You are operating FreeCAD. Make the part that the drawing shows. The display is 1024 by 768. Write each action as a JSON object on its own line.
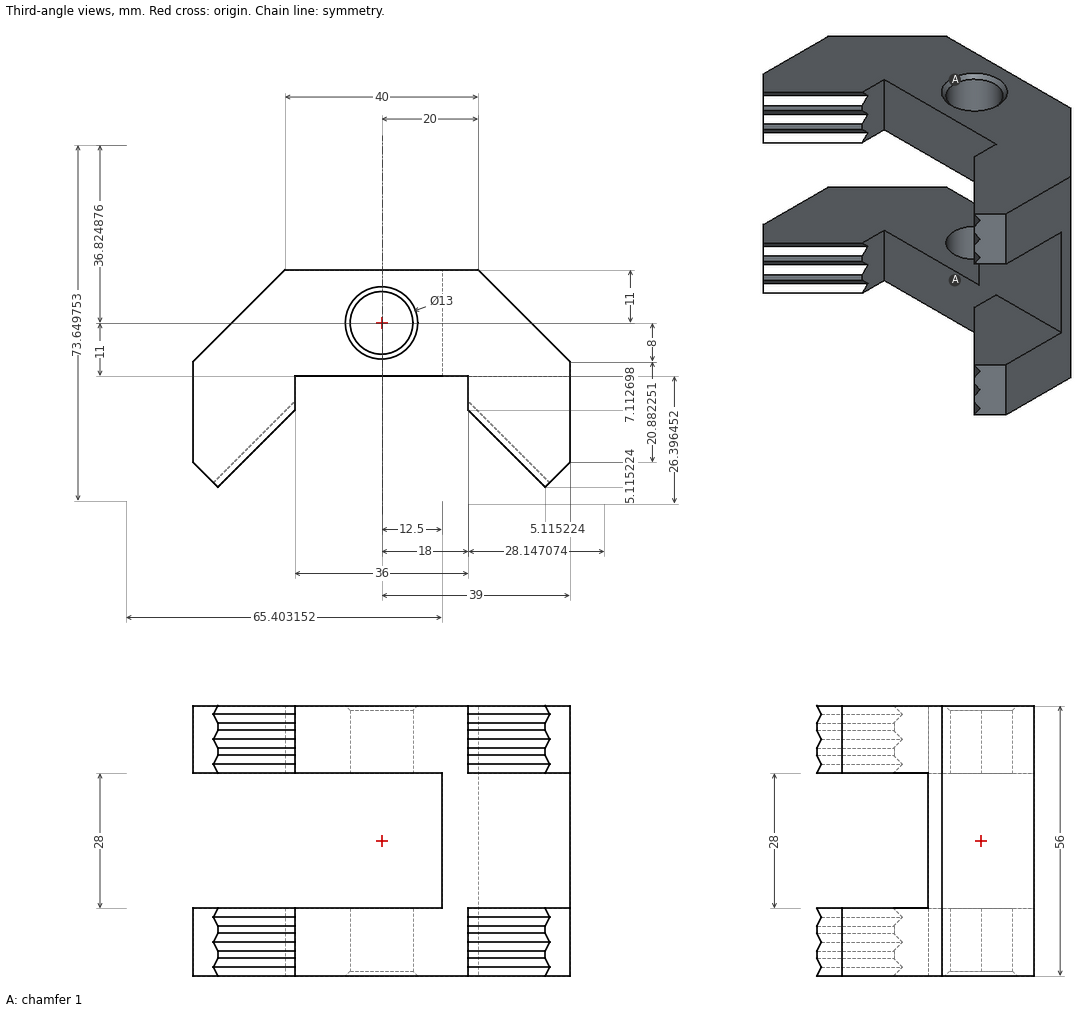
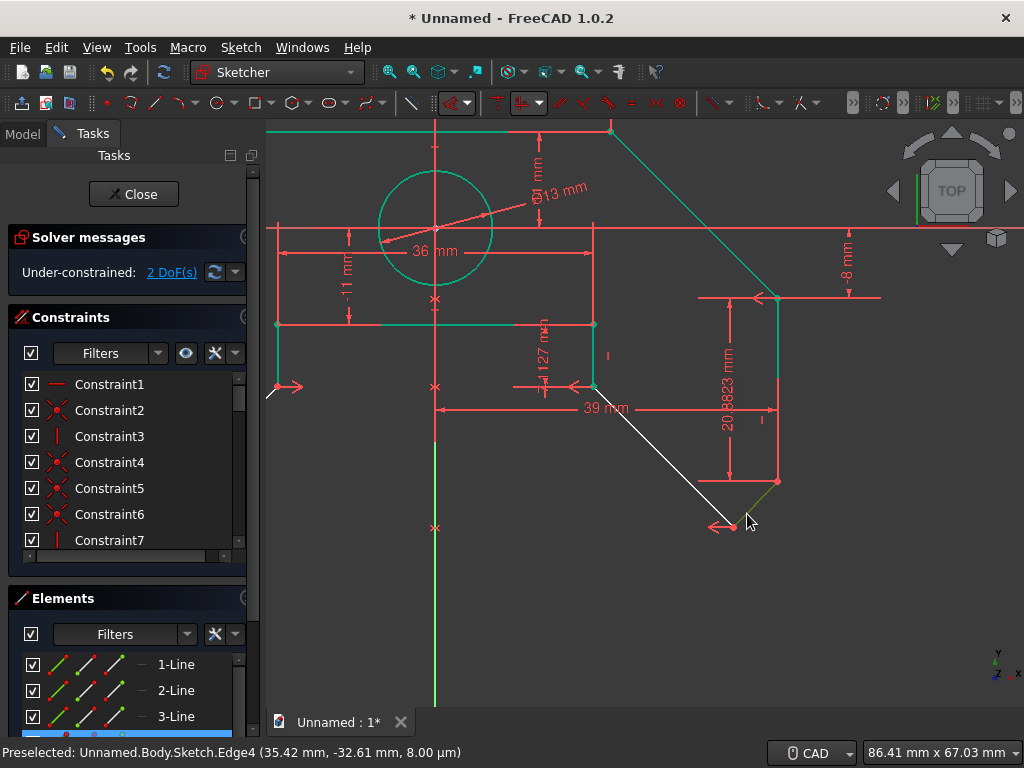
{"action": "key", "text": "l"}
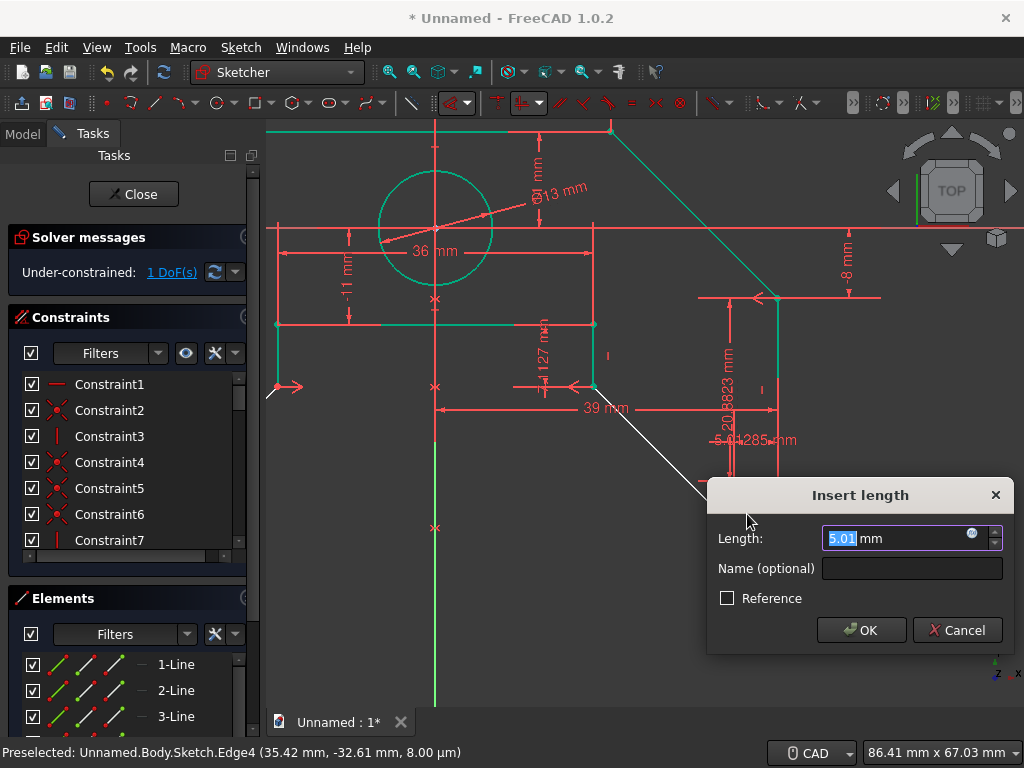
{"action": "type", "text": "5.115224"}
{"action": "key", "text": "Return"}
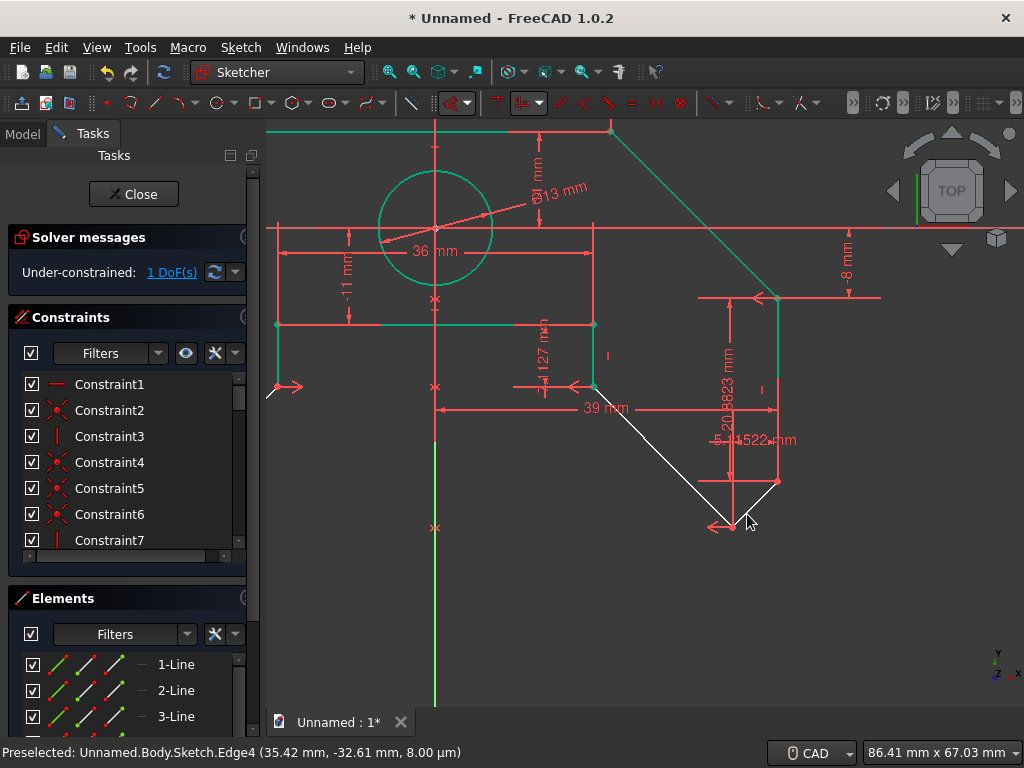
{"action": "left_click", "coordinate": [746, 514]}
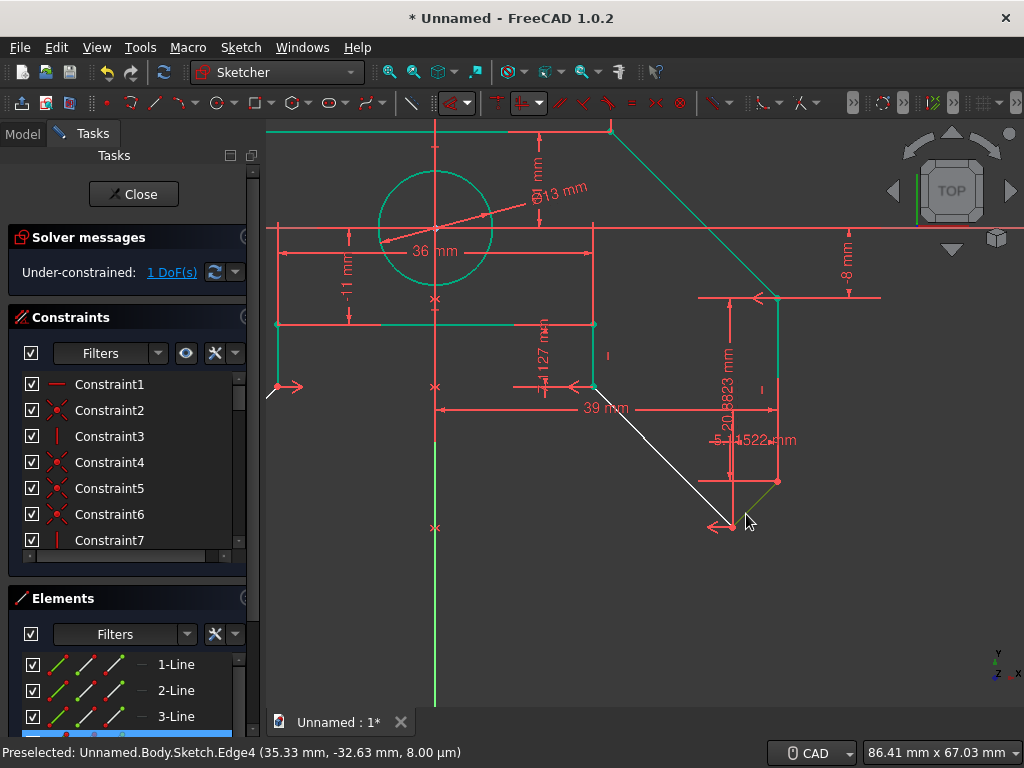
{"action": "left_click", "coordinate": [470, 104]}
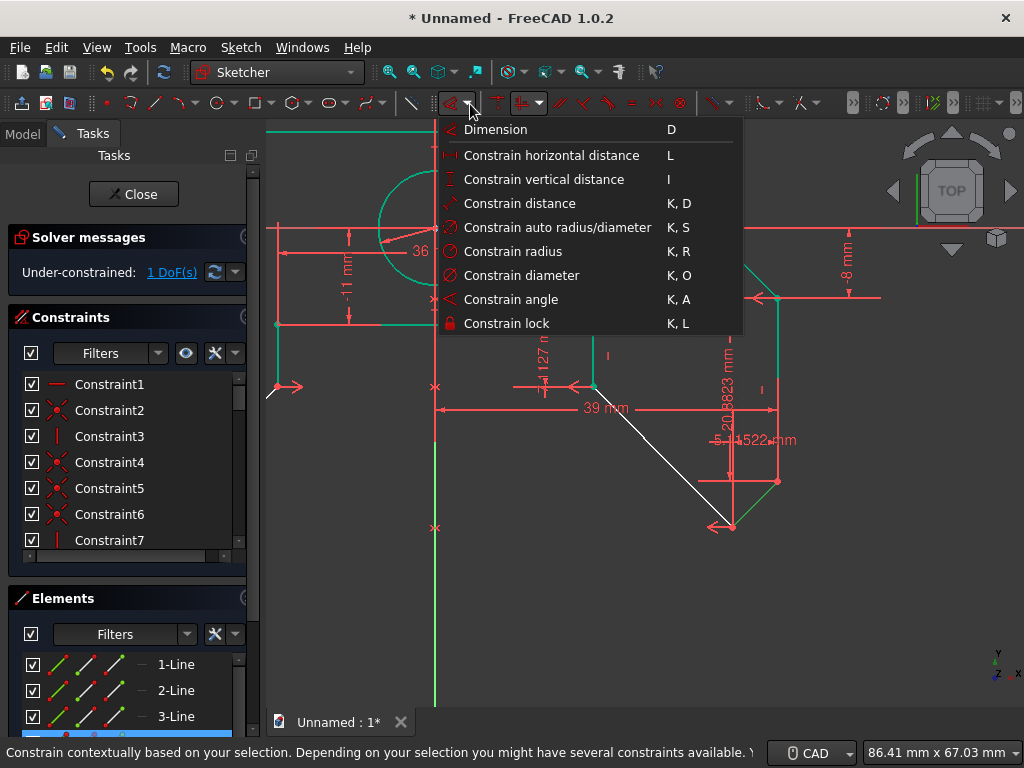
{"action": "left_click", "coordinate": [591, 179]}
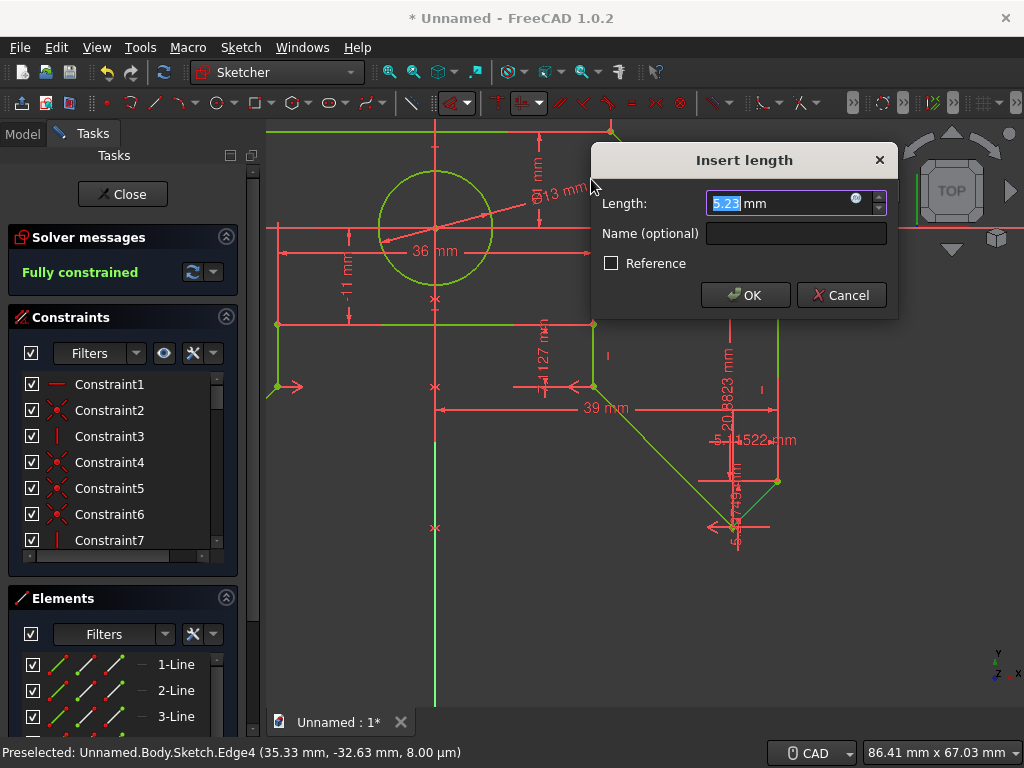
{"action": "type", "text": "5.115224"}
{"action": "key", "text": "Return"}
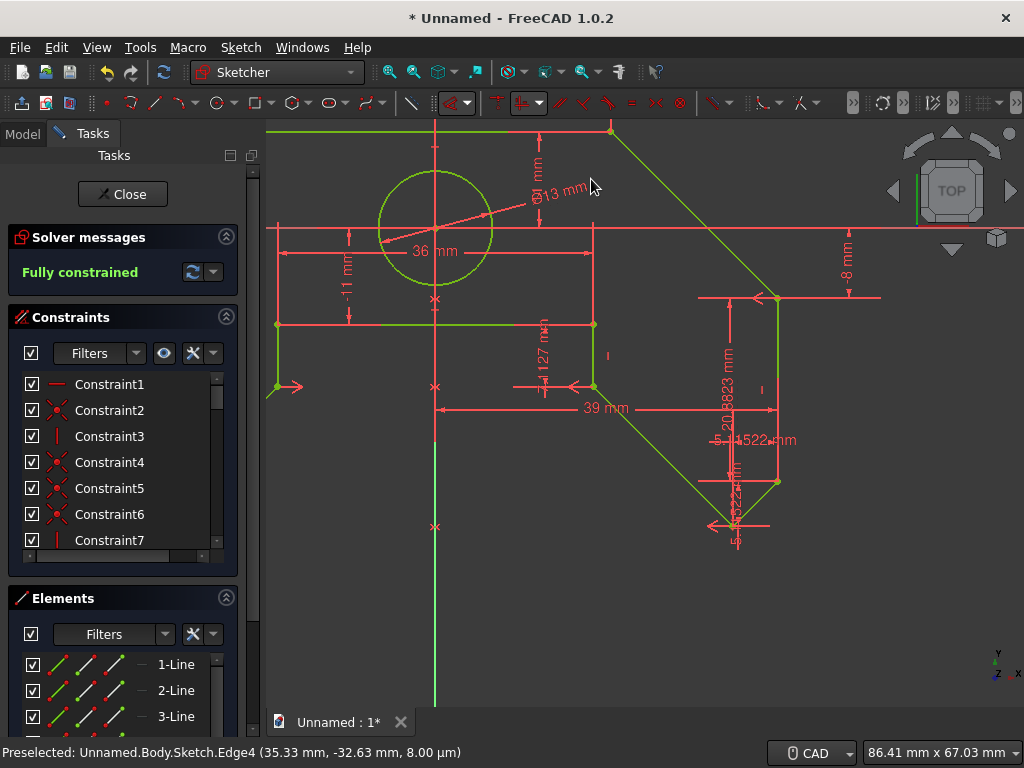
{"action": "left_click", "coordinate": [123, 194]}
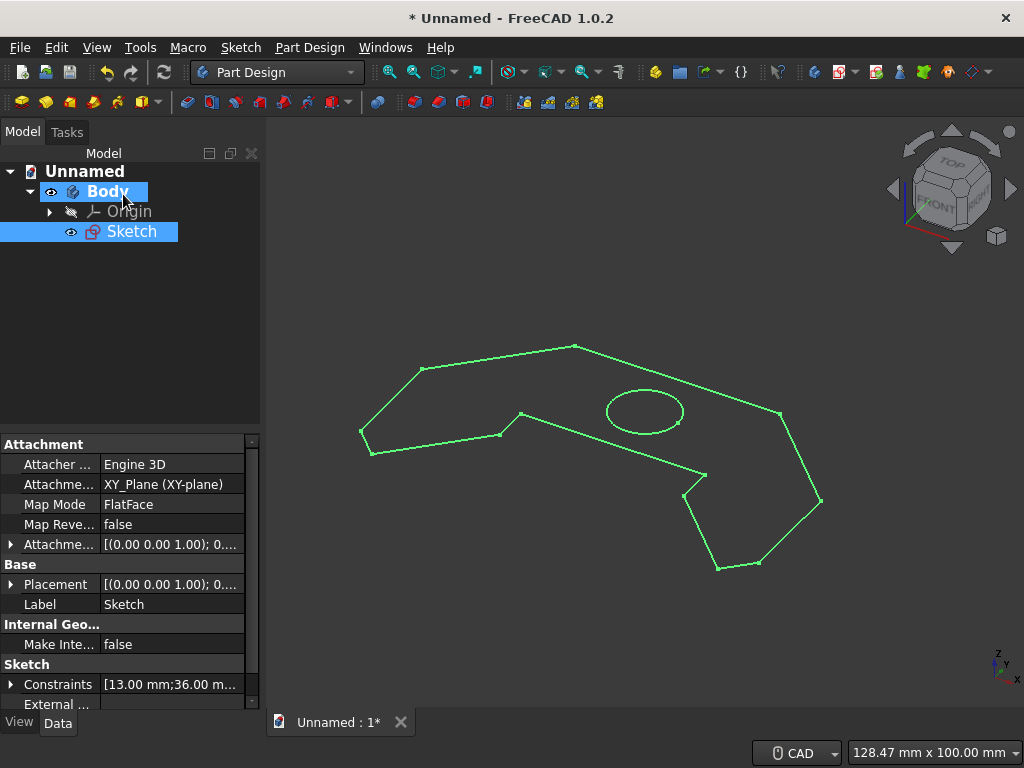
{"action": "left_click", "coordinate": [22, 102]}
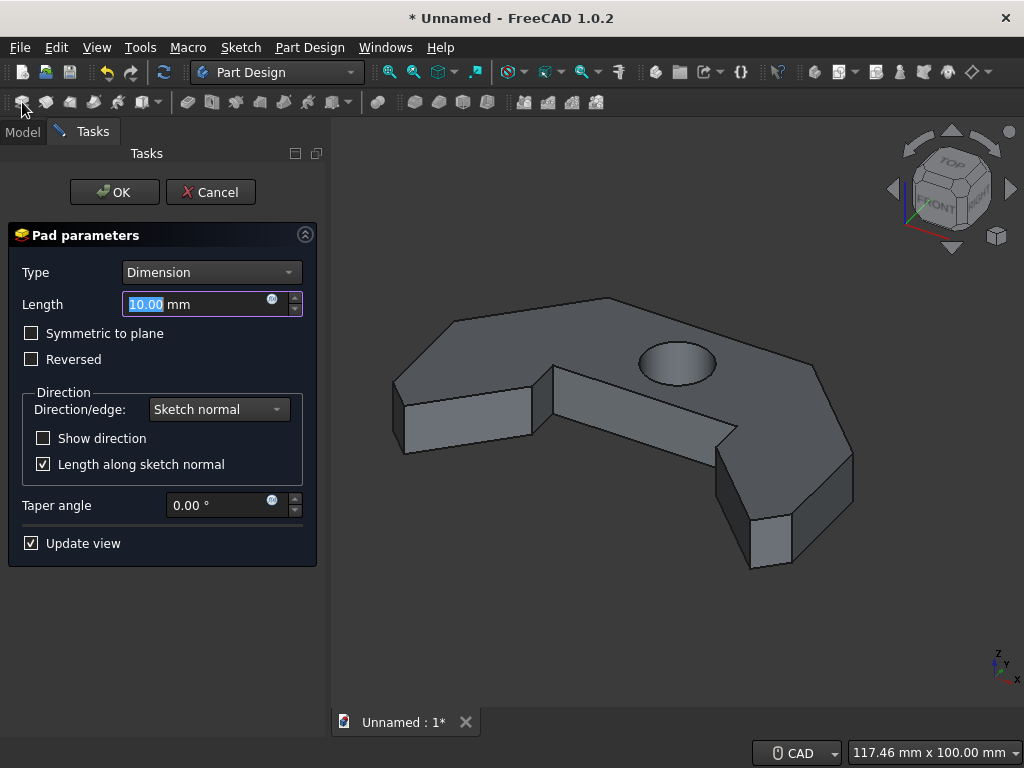
{"action": "type", "text": "56"}
{"action": "key", "text": "Tab"}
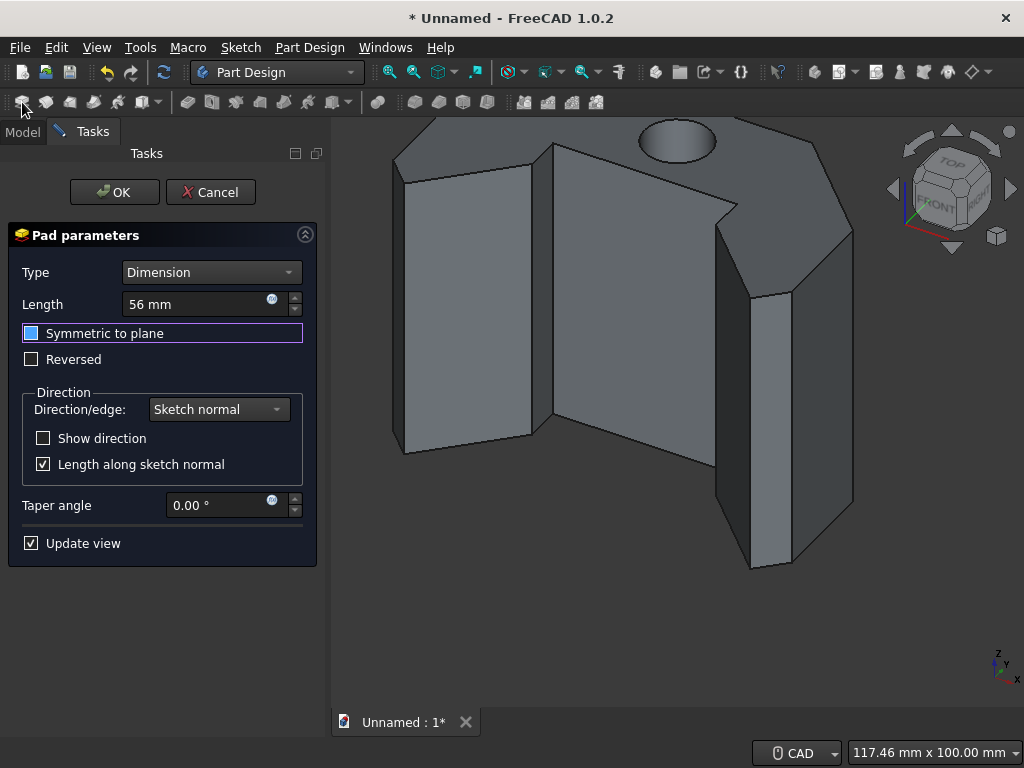
{"action": "left_click", "coordinate": [30, 333]}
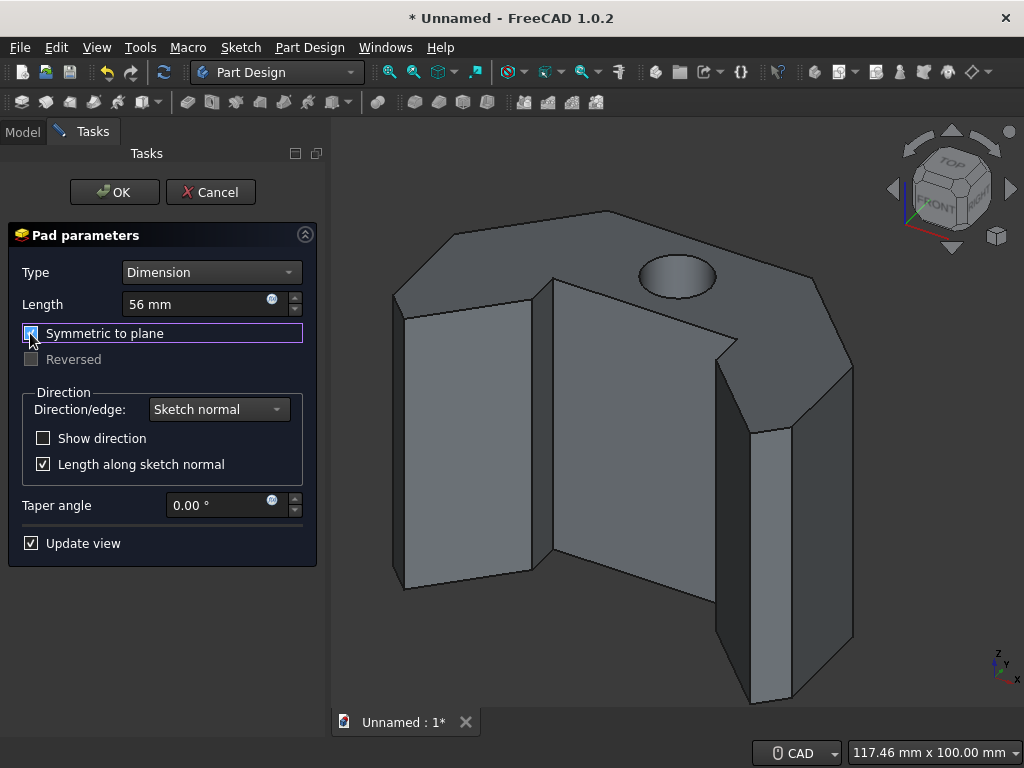
{"action": "left_click", "coordinate": [115, 192]}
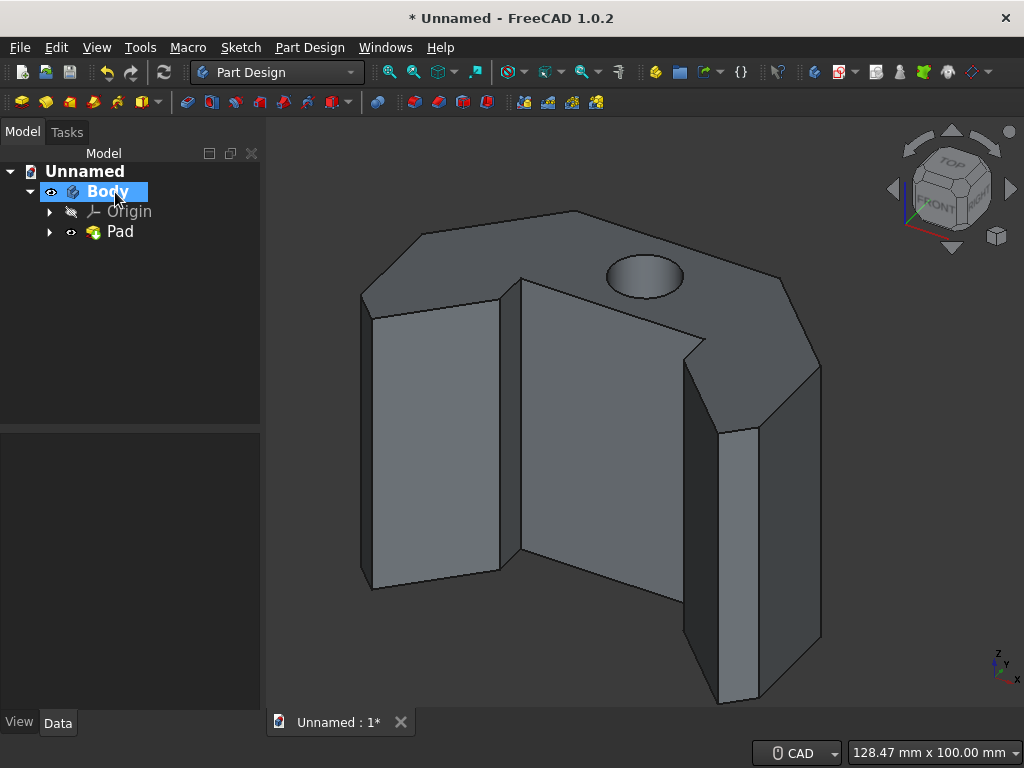
{"action": "left_click", "coordinate": [390, 72]}